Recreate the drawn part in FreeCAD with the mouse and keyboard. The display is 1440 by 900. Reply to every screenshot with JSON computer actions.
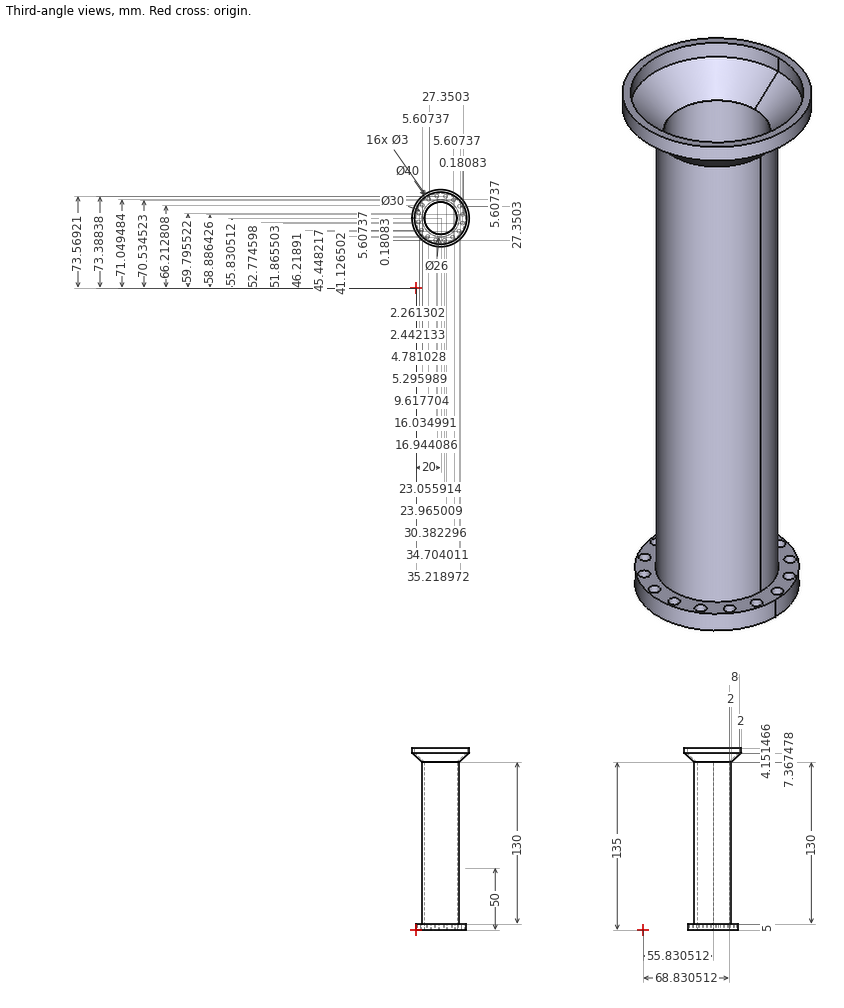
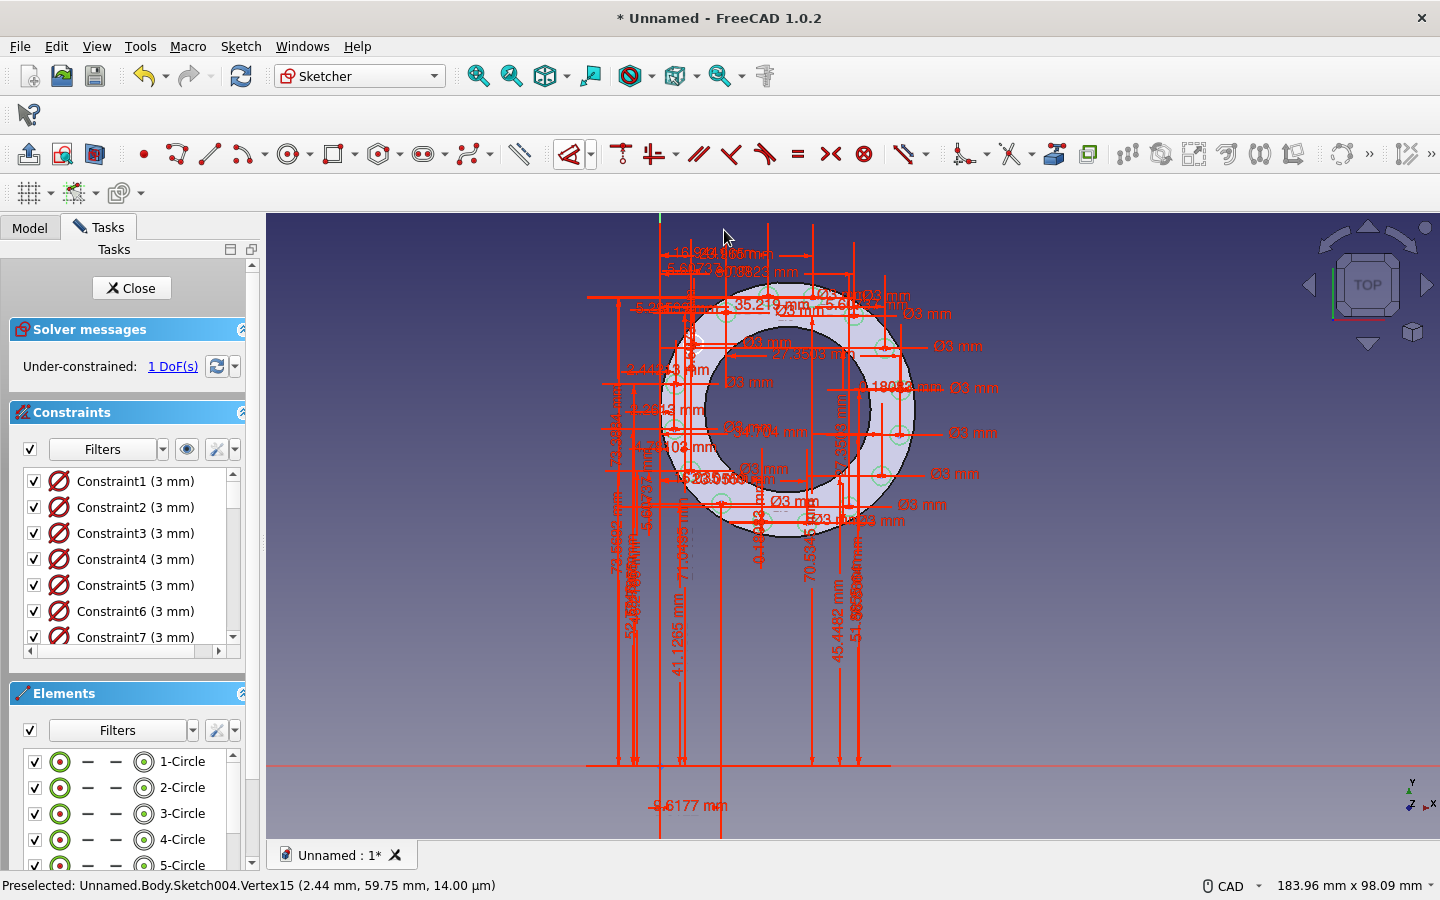
{"action": "left_click", "coordinate": [694, 344]}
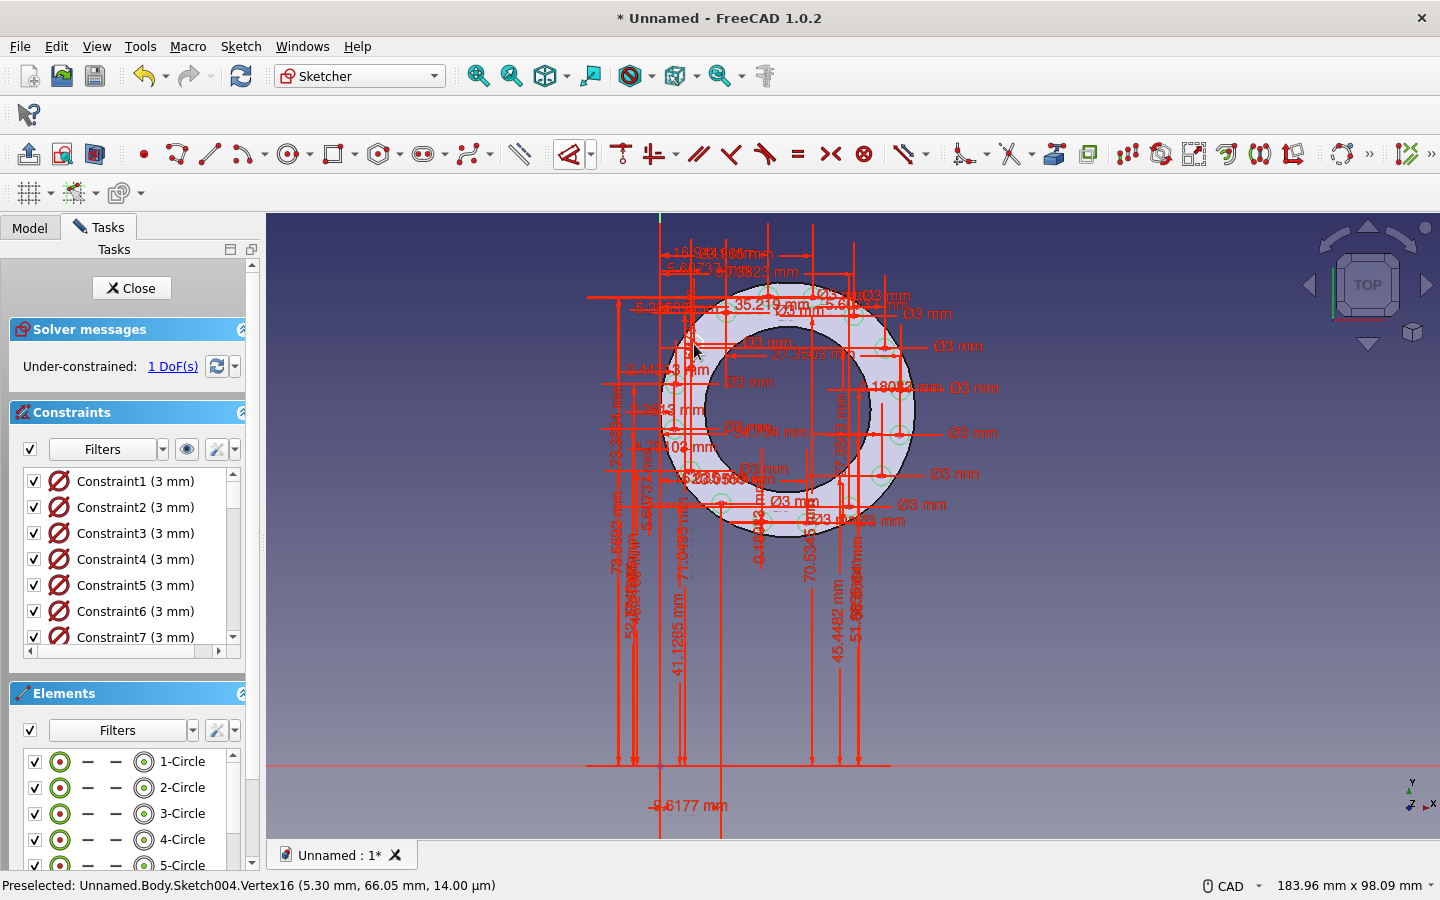
{"action": "key", "text": "i"}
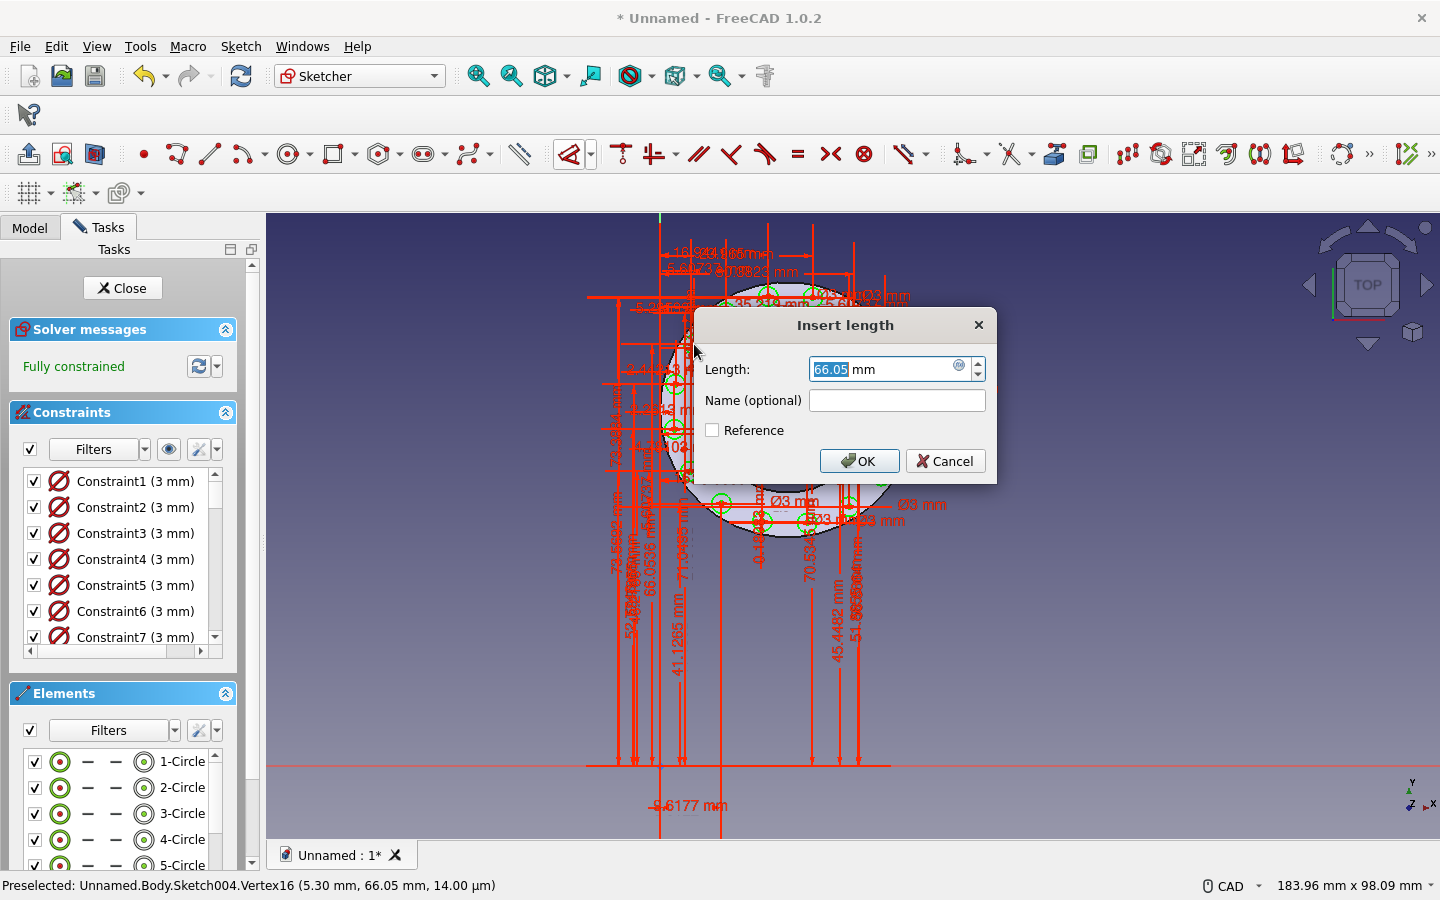
{"action": "type", "text": "66.212808"}
{"action": "key", "text": "Return"}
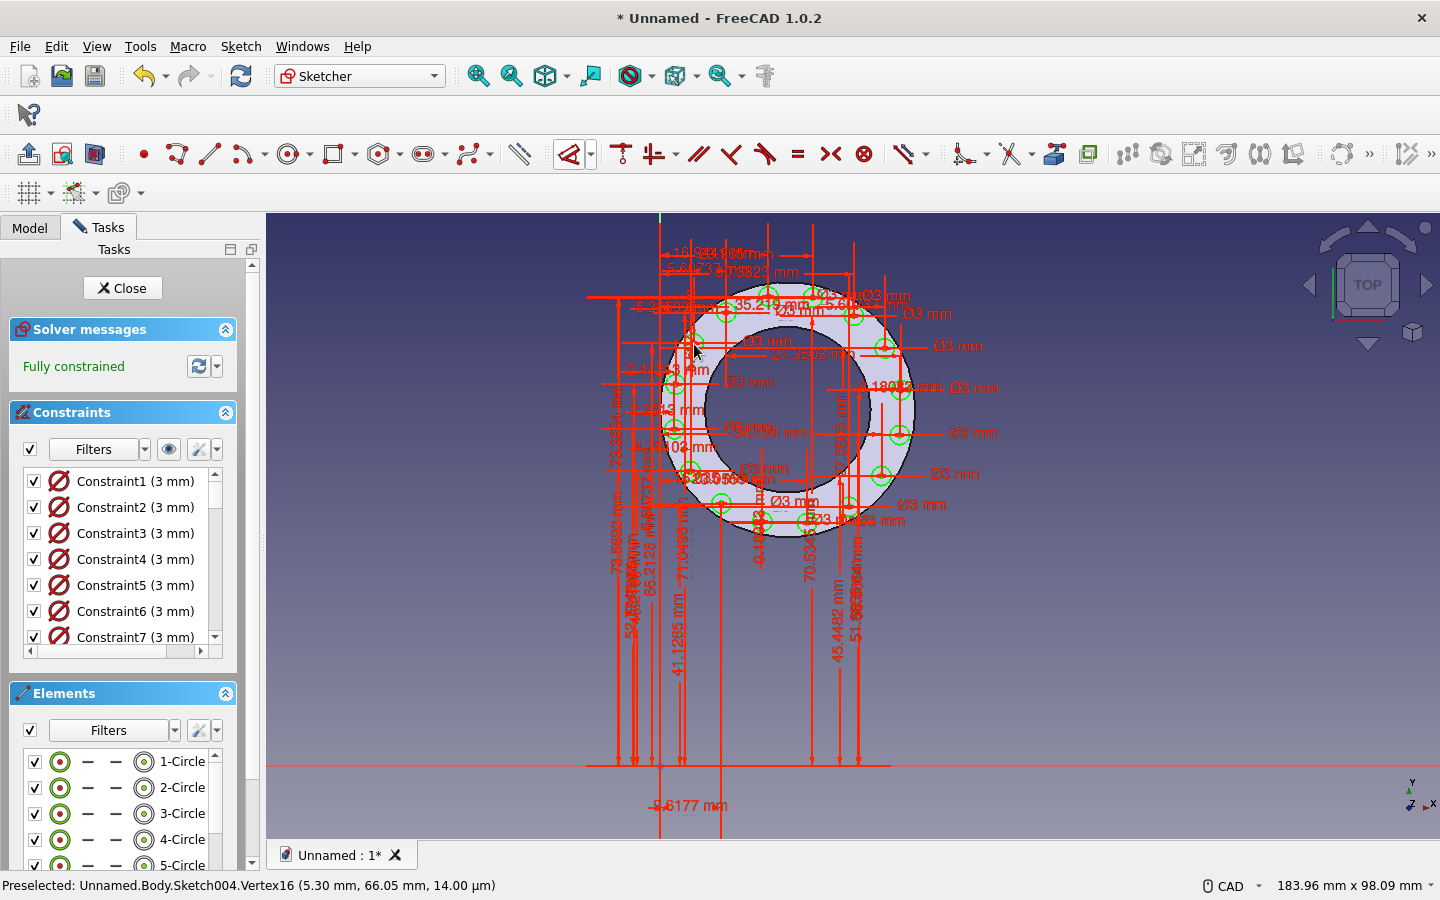
{"action": "left_click", "coordinate": [123, 288]}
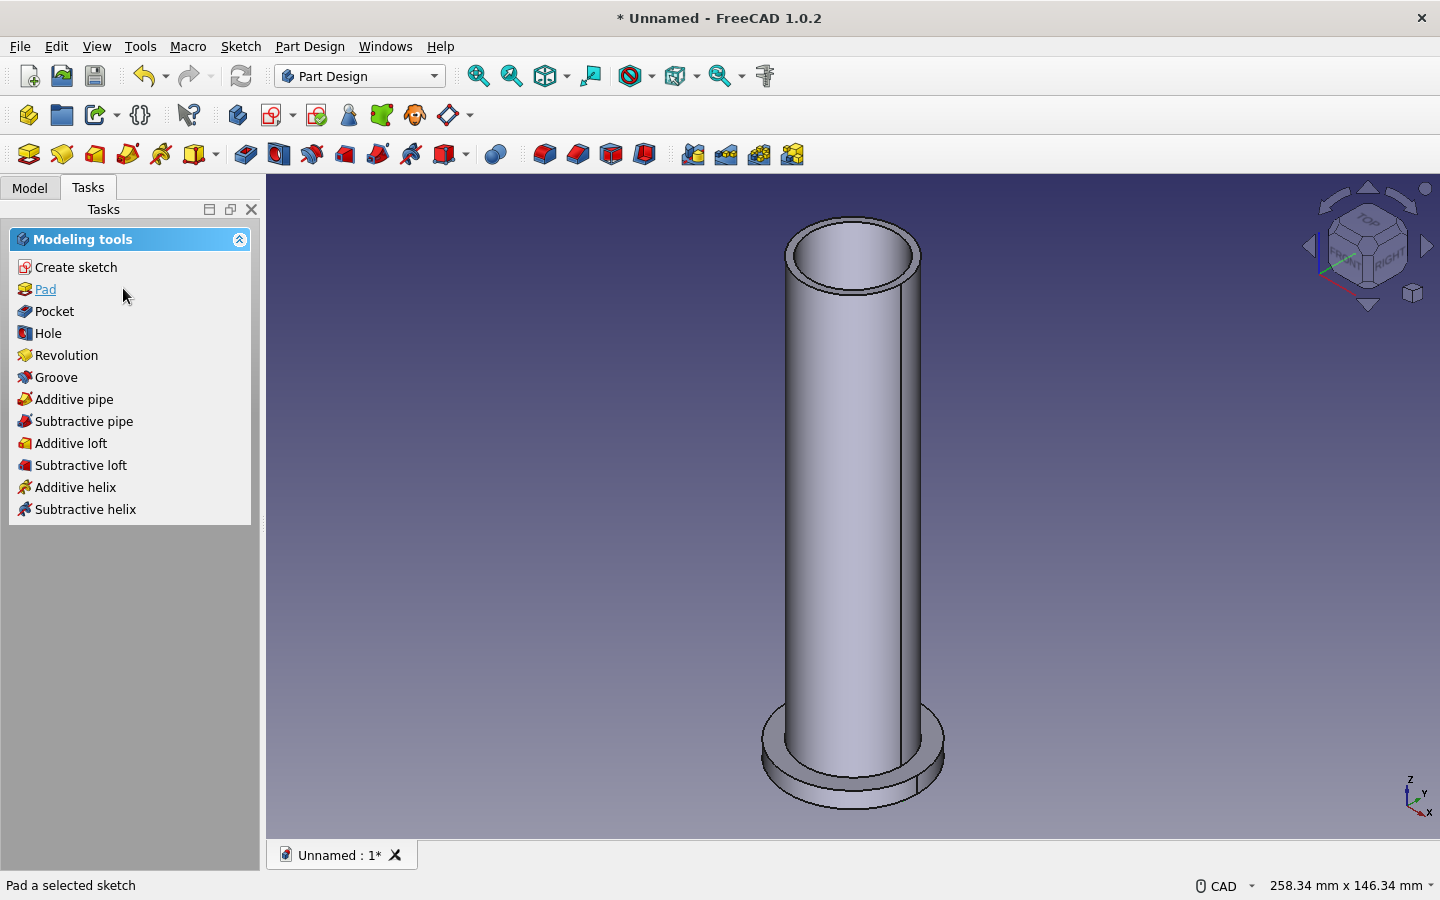
{"action": "left_click", "coordinate": [246, 154]}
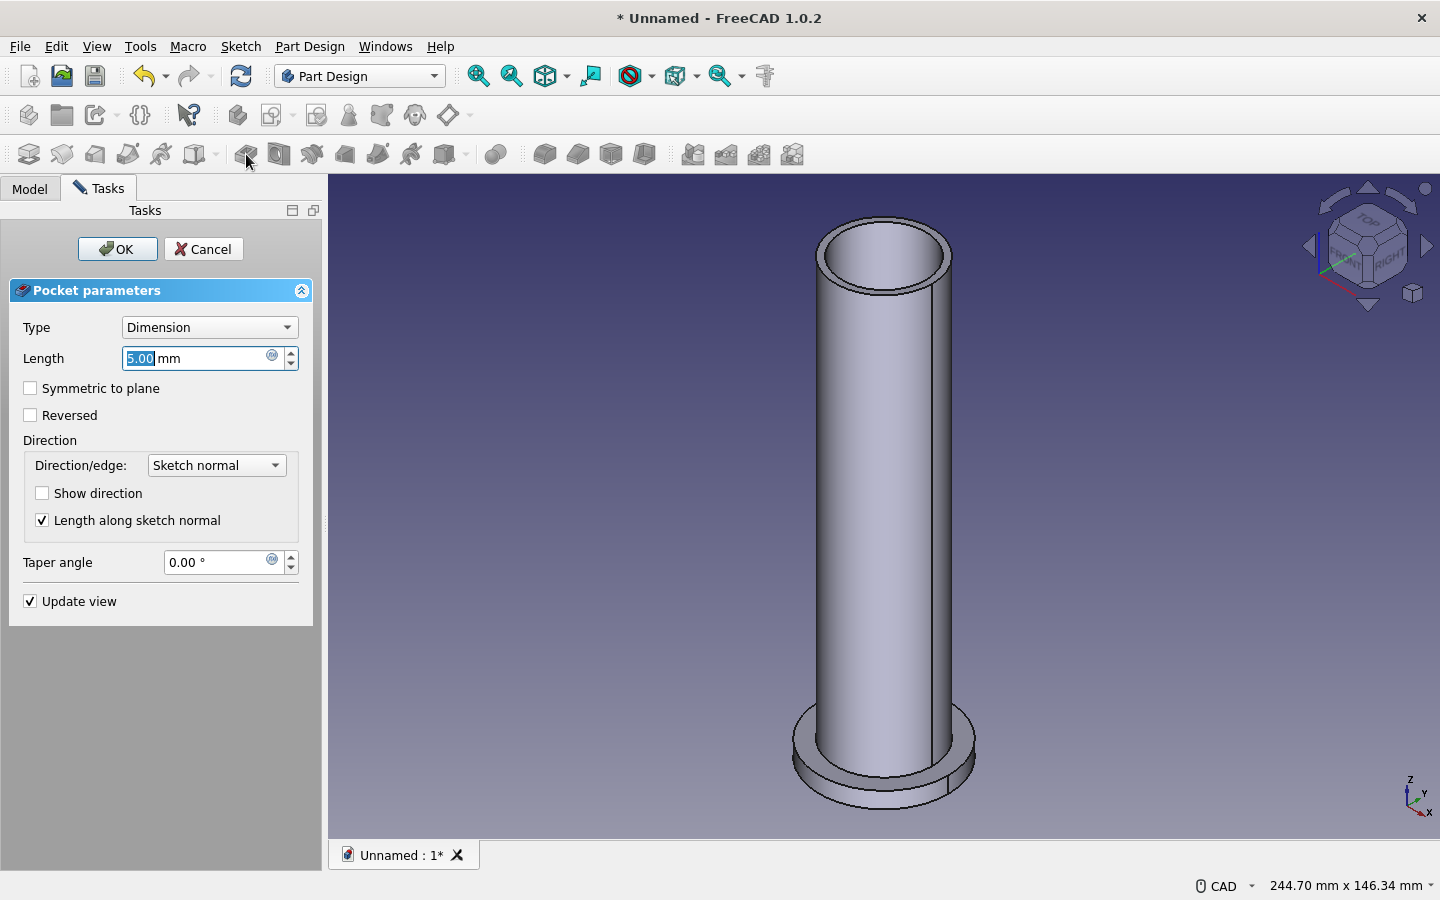
{"action": "type", "text": "50"}
{"action": "key", "text": "Tab"}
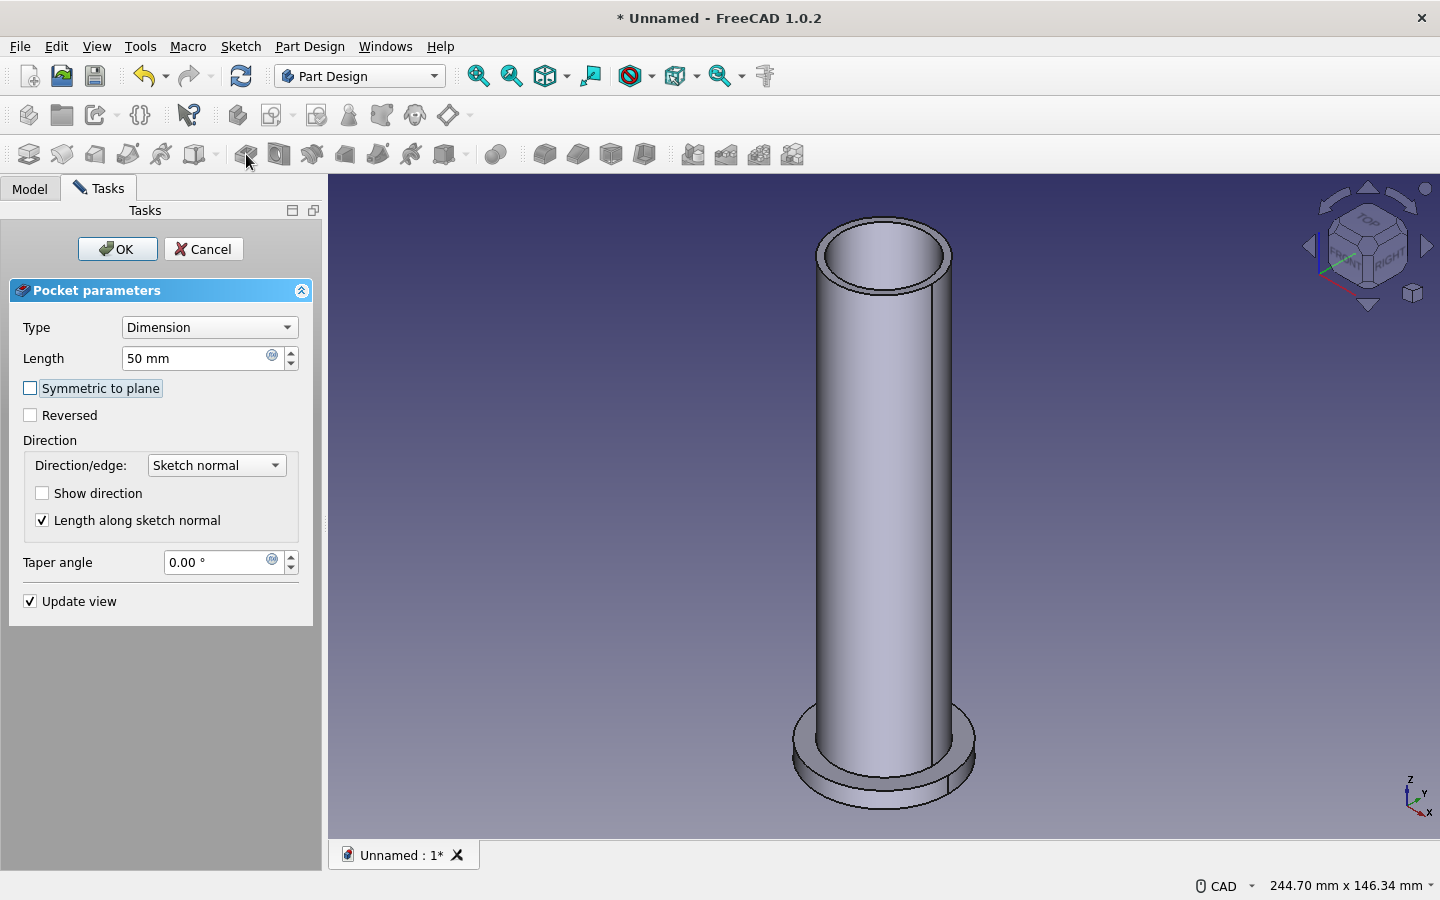
{"action": "left_click", "coordinate": [31, 415]}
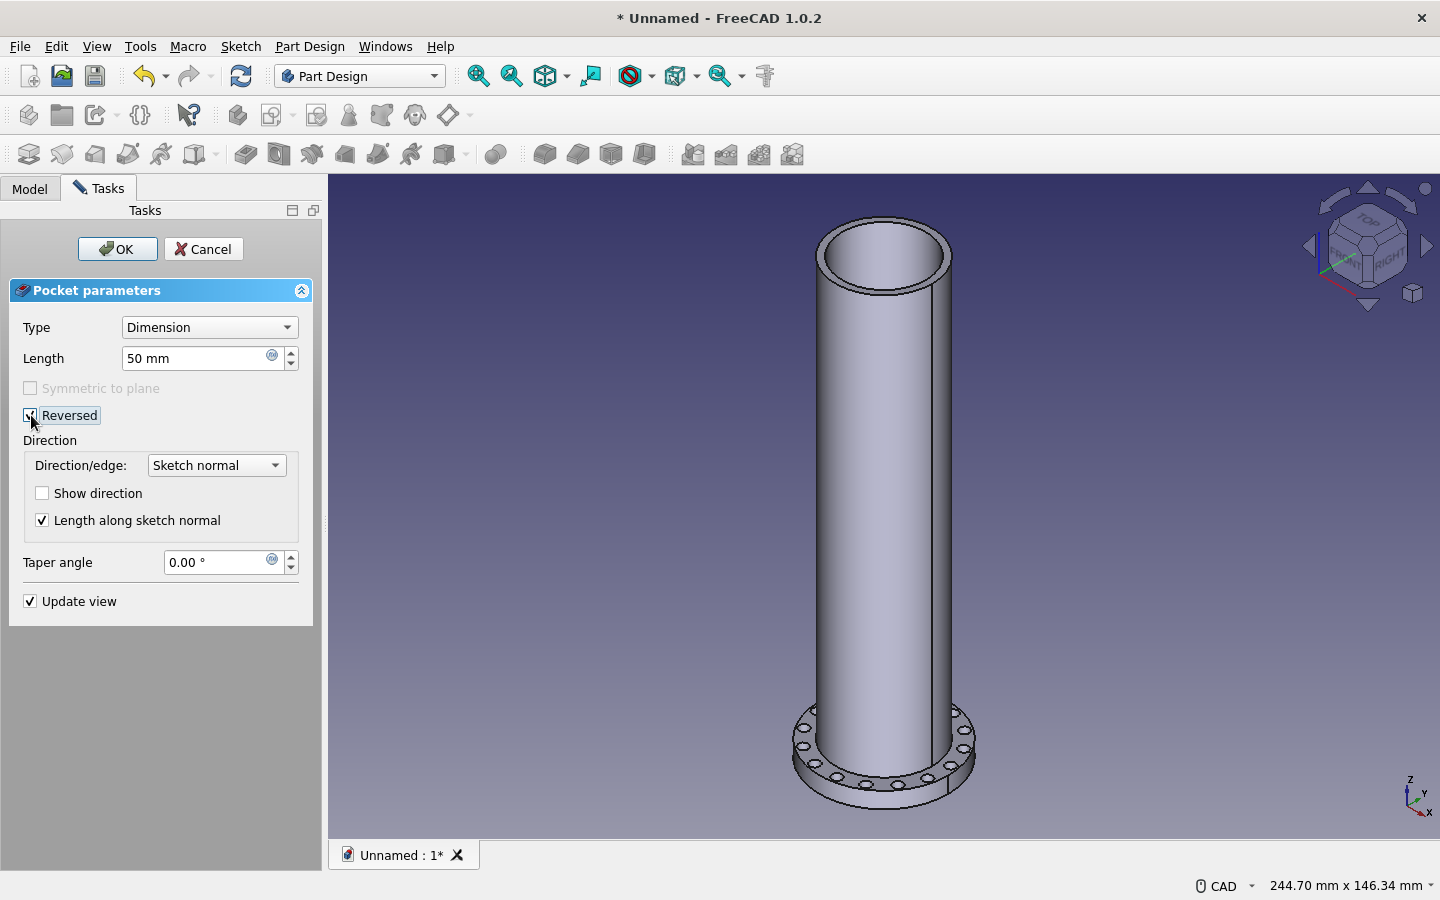
{"action": "left_click", "coordinate": [118, 249]}